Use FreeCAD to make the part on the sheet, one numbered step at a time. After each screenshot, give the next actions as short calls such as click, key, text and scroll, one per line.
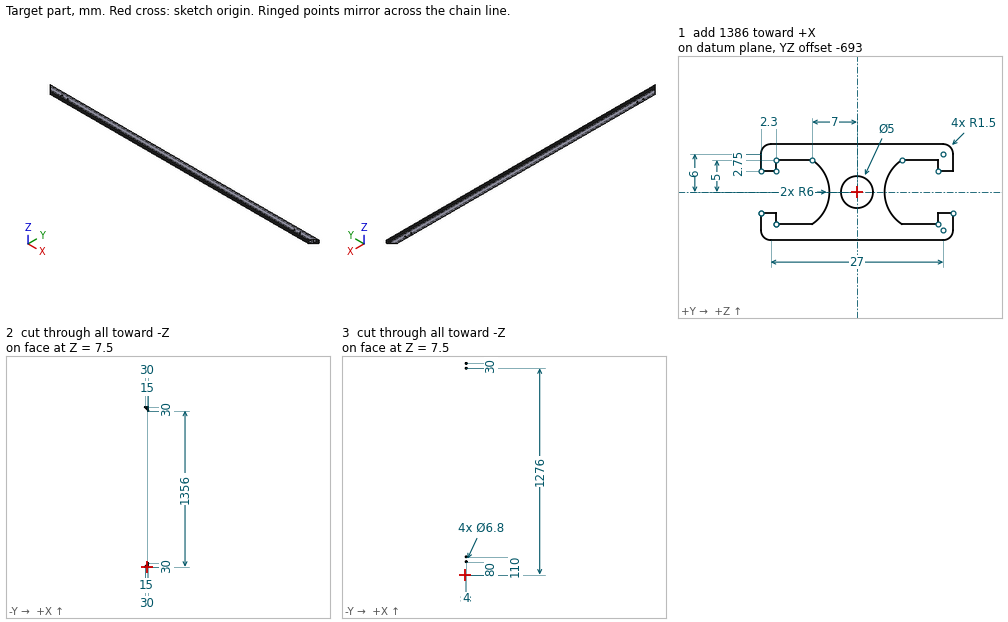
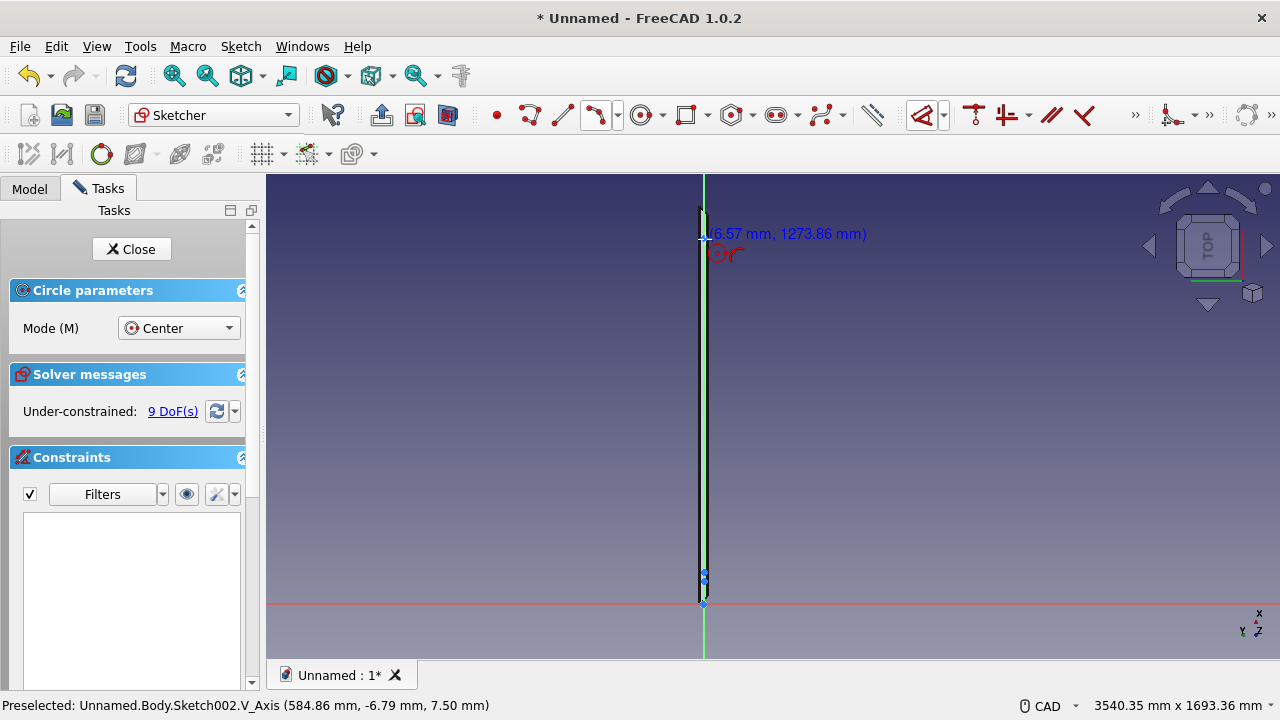
scroll(705, 230, up, 16)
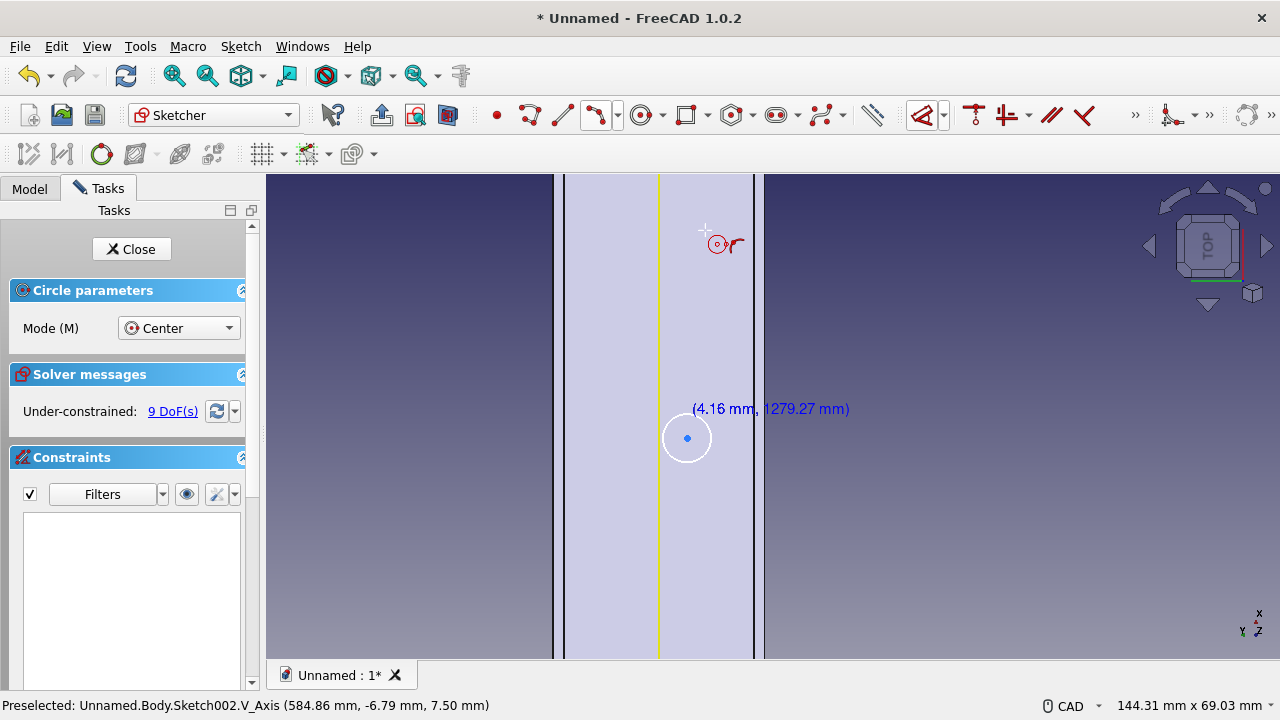
click(687, 226)
click(704, 209)
key(Escape)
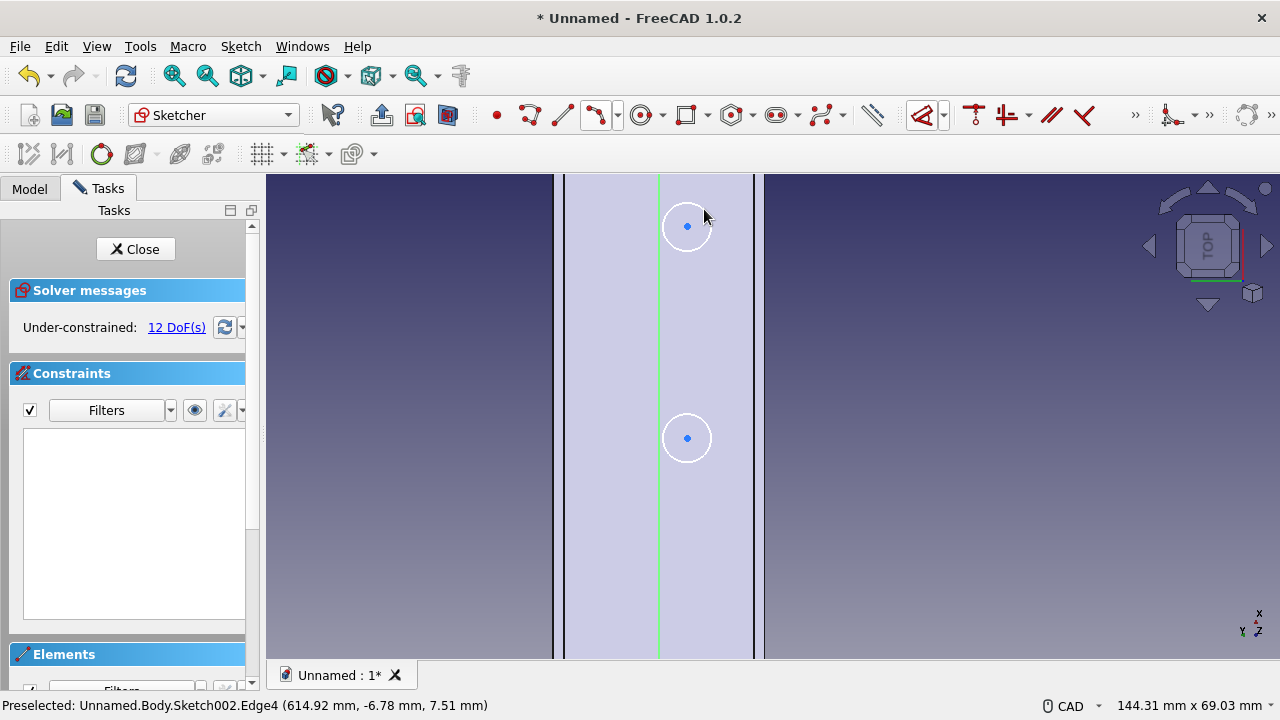
scroll(705, 230, down, 16)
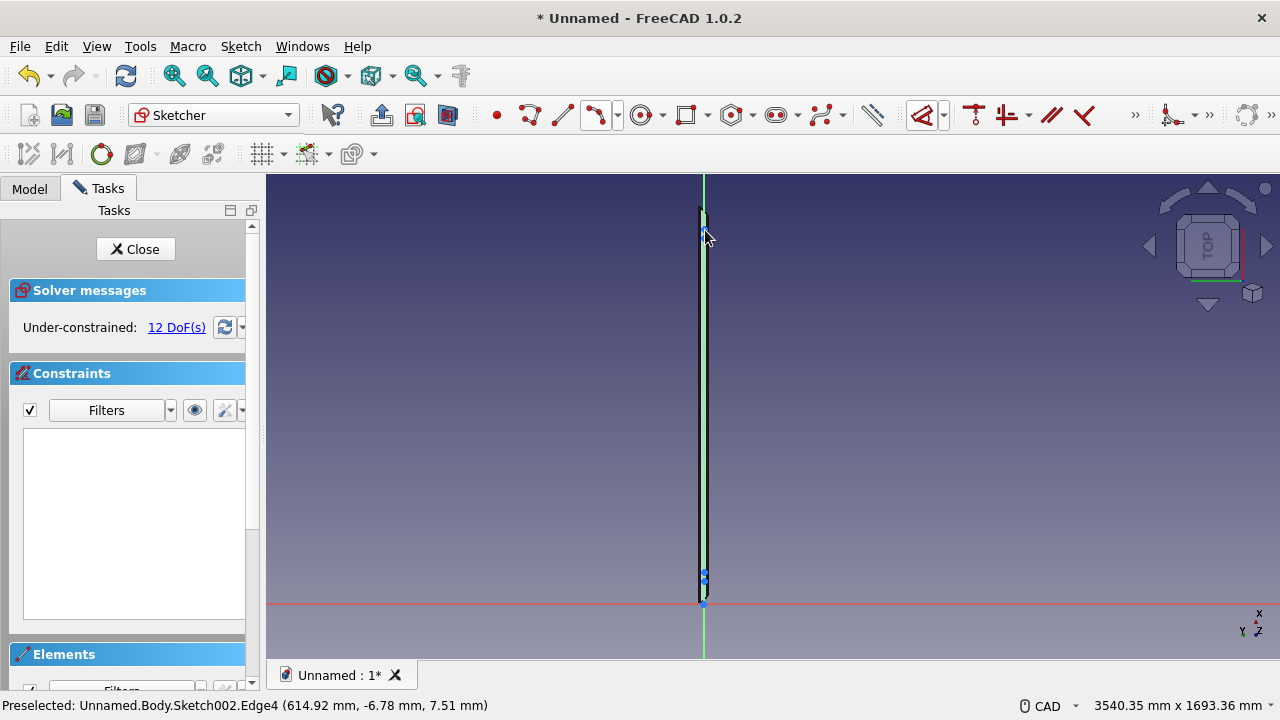
scroll(705, 580, up, 13)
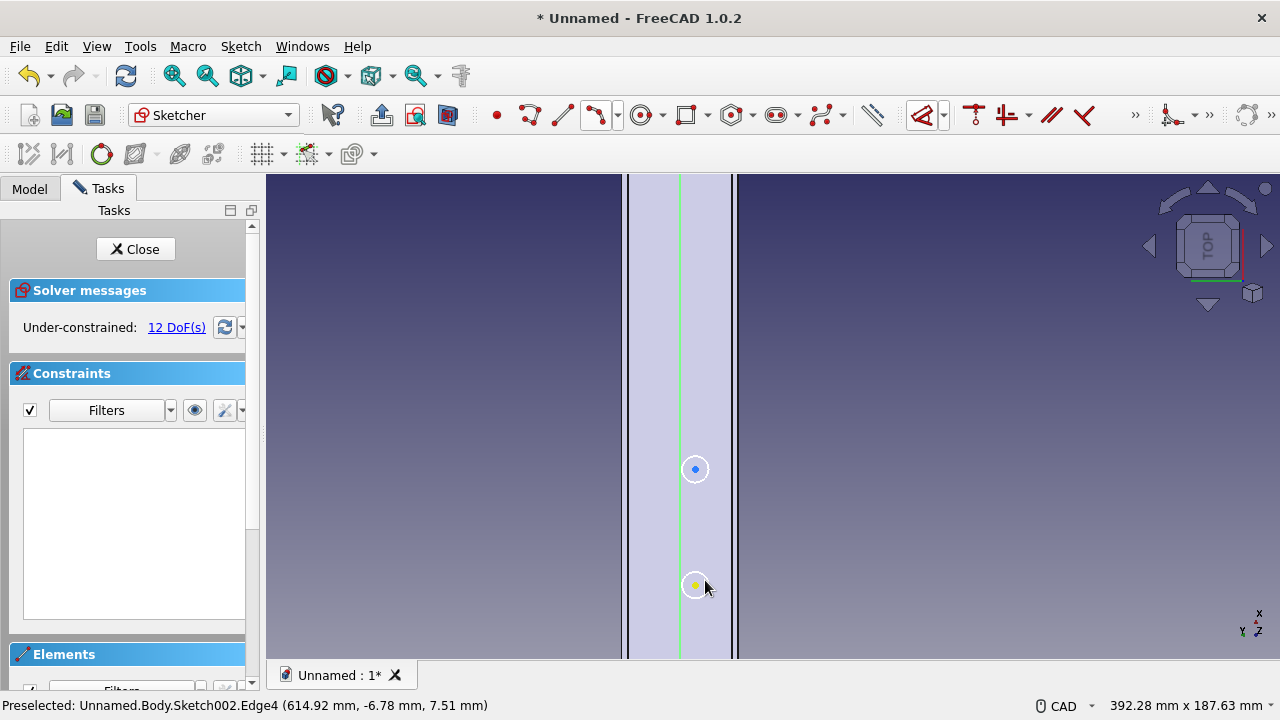
click(705, 576)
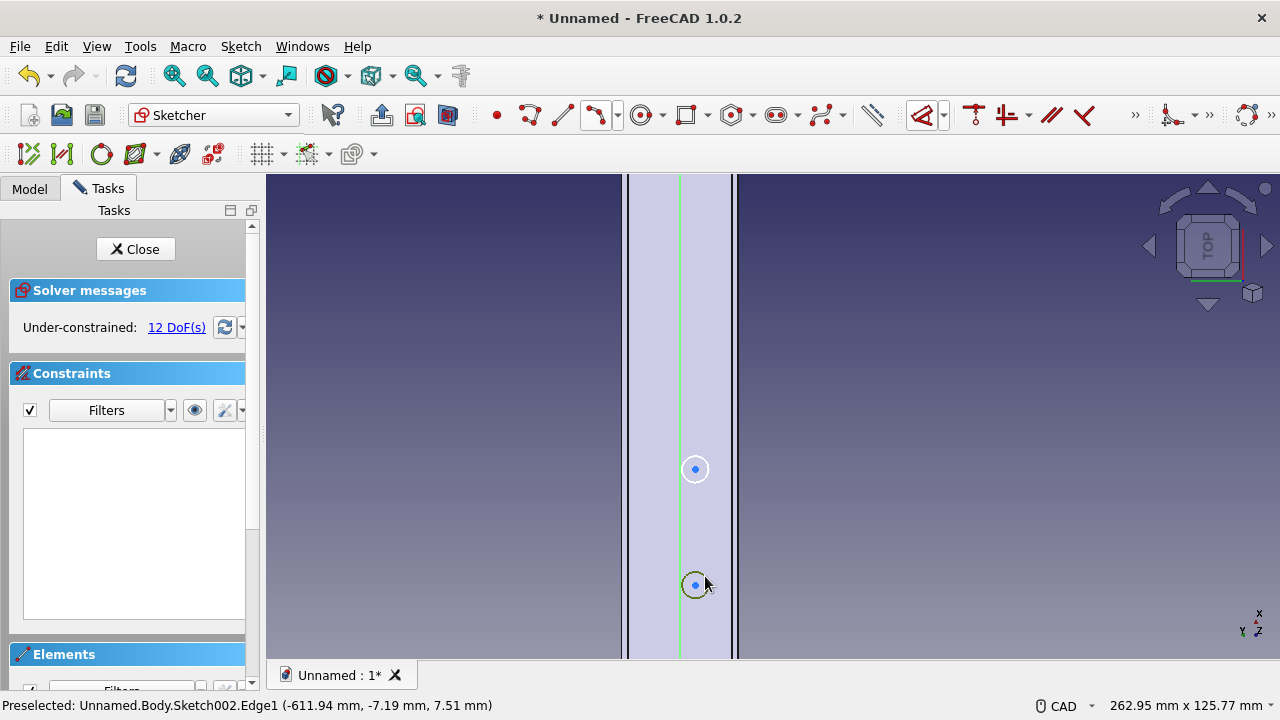
click(705, 460)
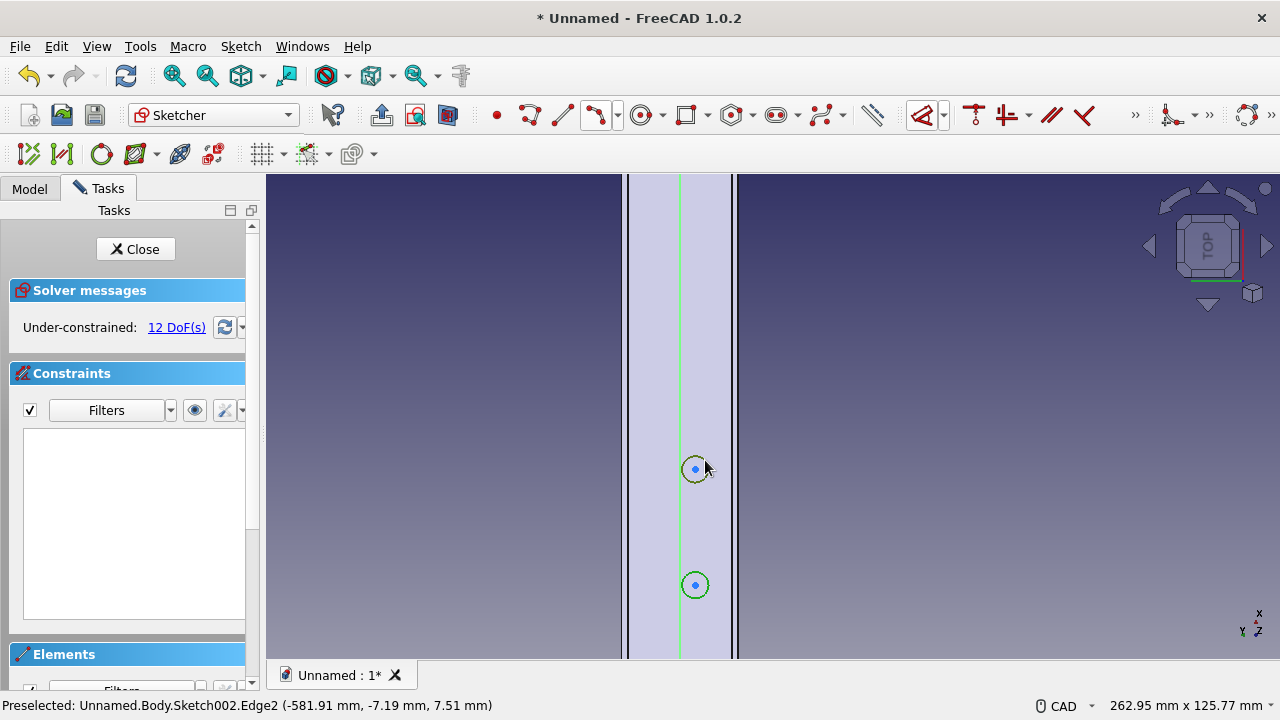
scroll(705, 549, down, 14)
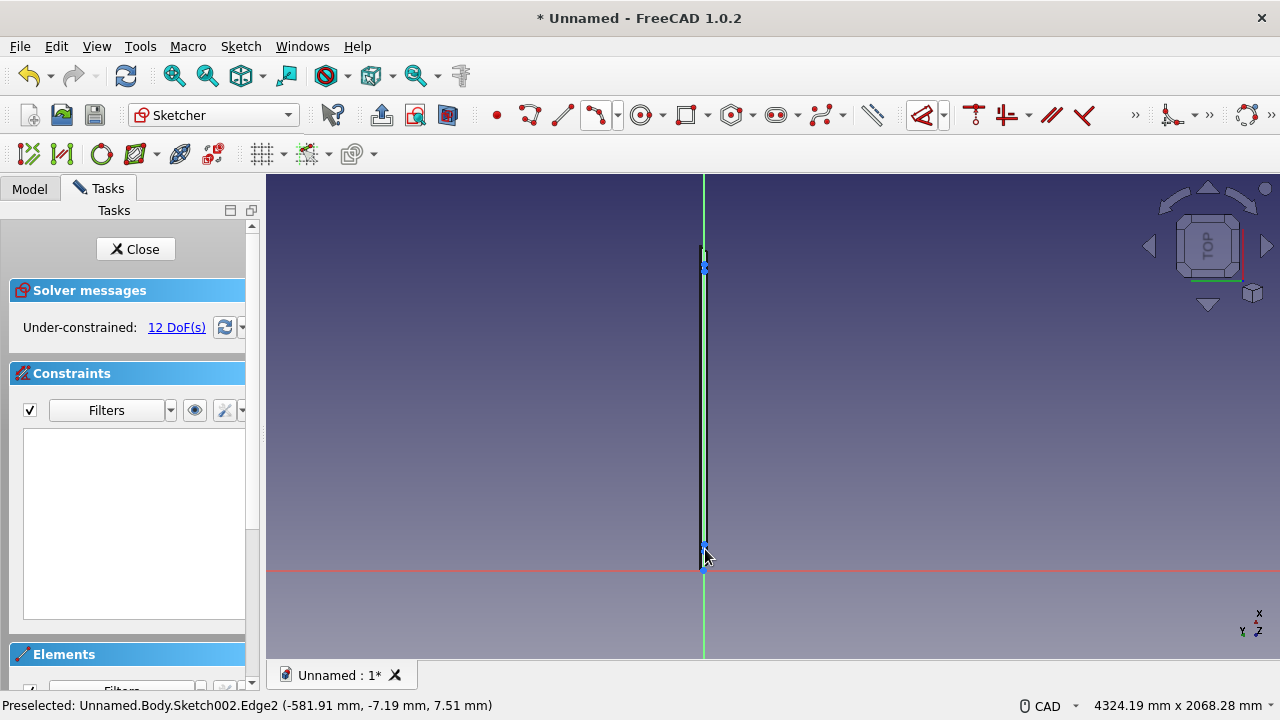
scroll(705, 271, up, 14)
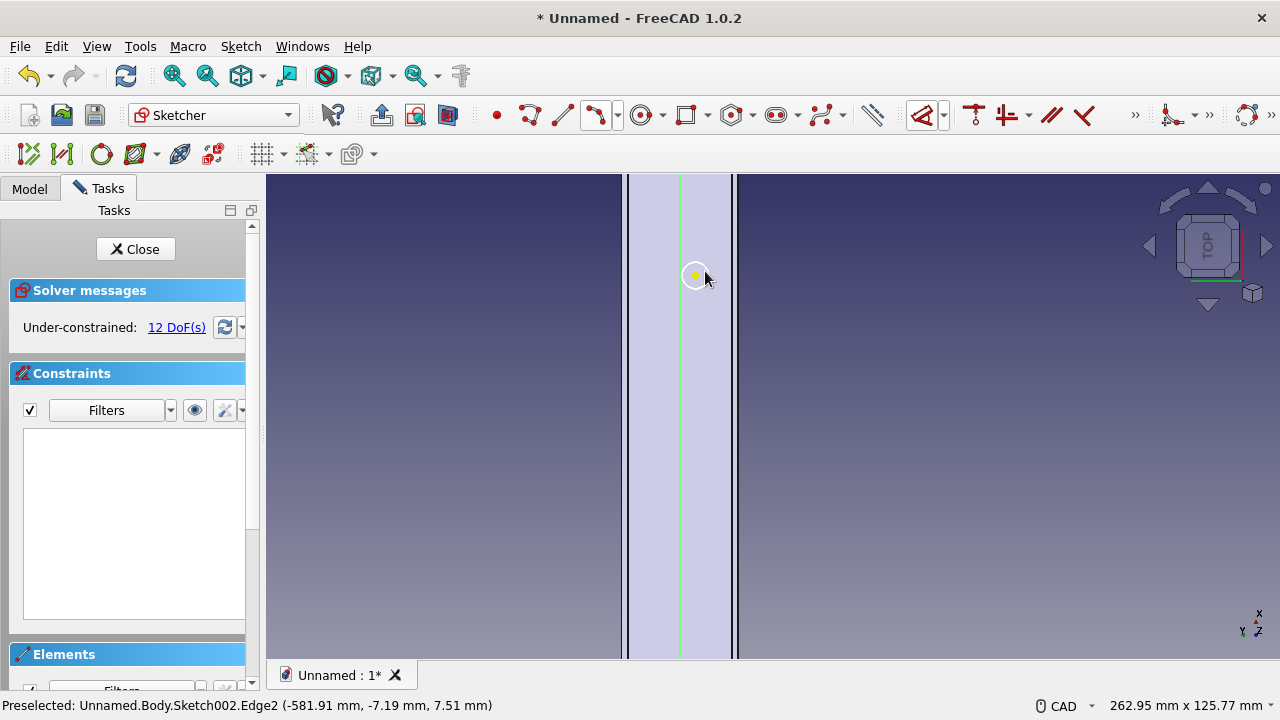
click(705, 266)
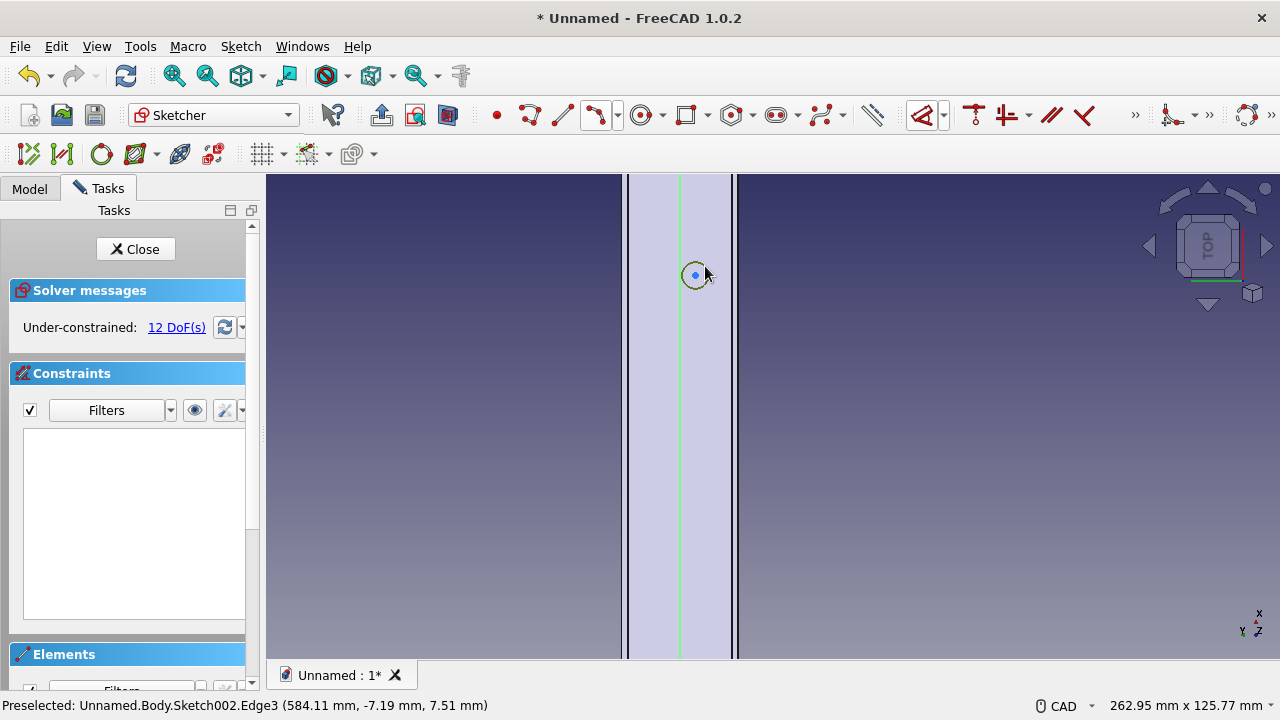
scroll(705, 271, down, 14)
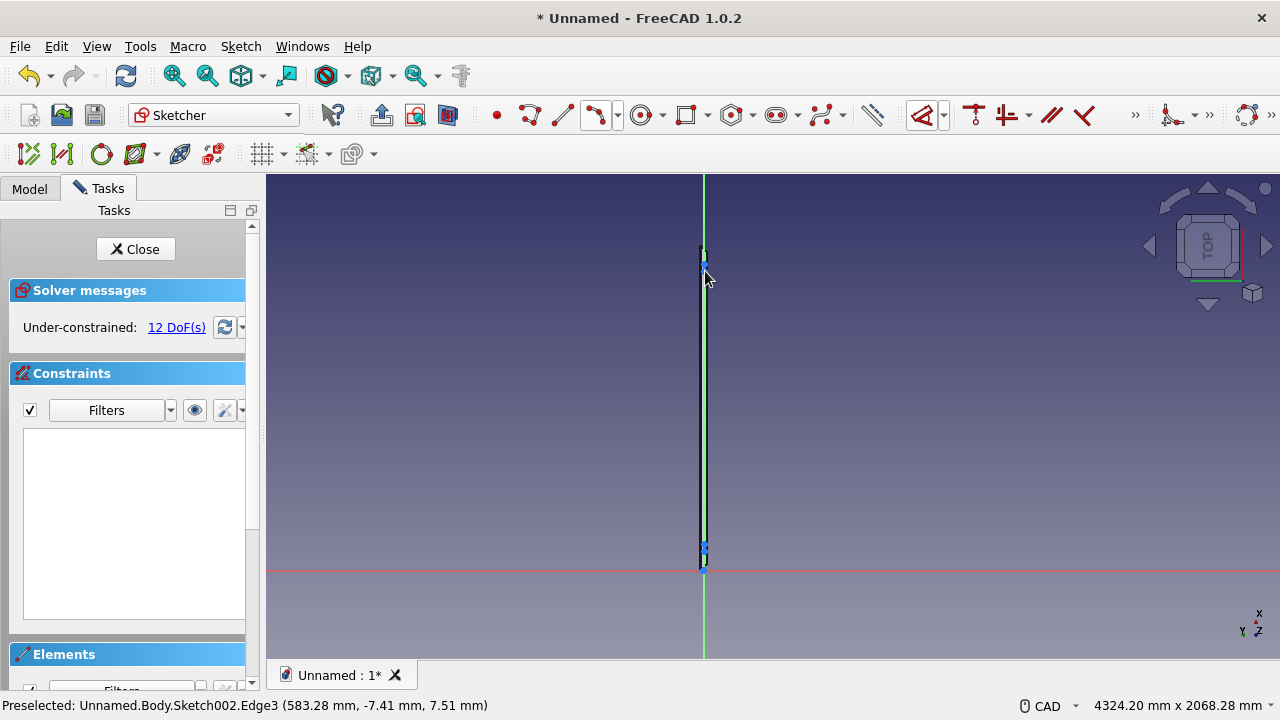
scroll(705, 264, up, 14)